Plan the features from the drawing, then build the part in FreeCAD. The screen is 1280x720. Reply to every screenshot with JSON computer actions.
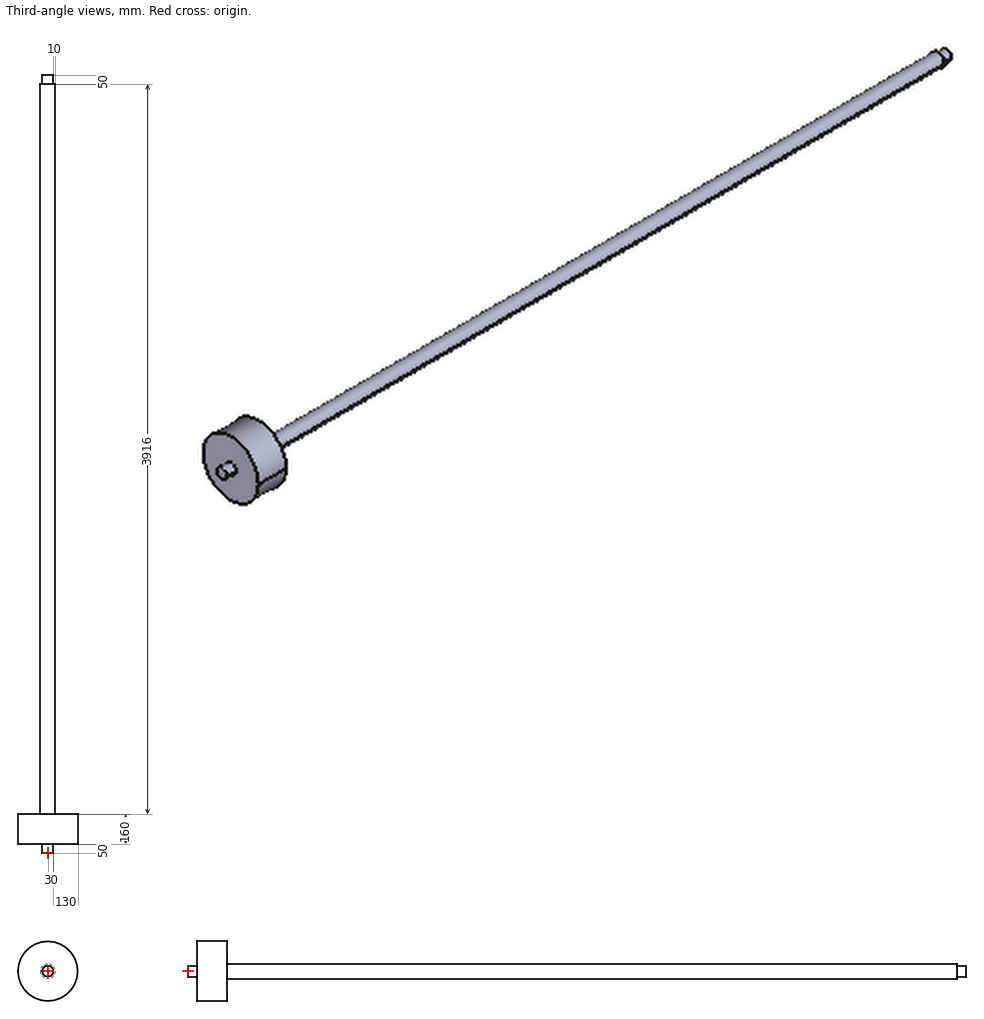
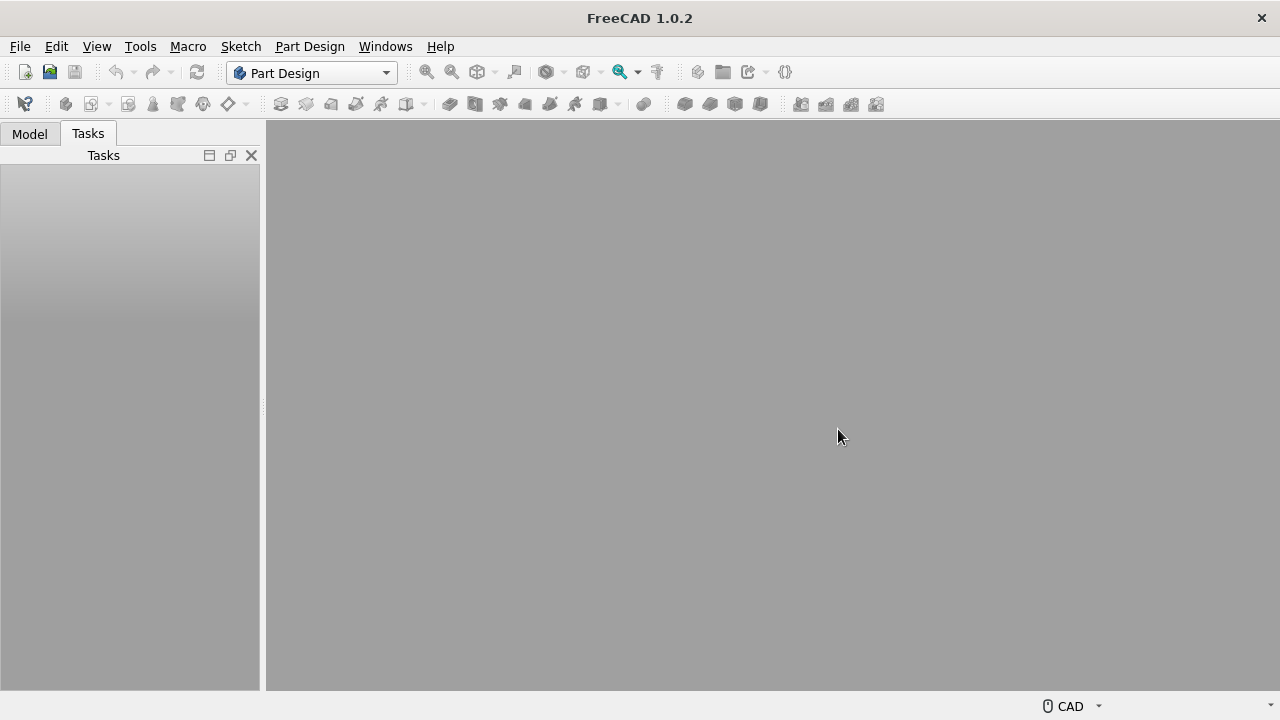
{"action": "left_click", "coordinate": [25, 72]}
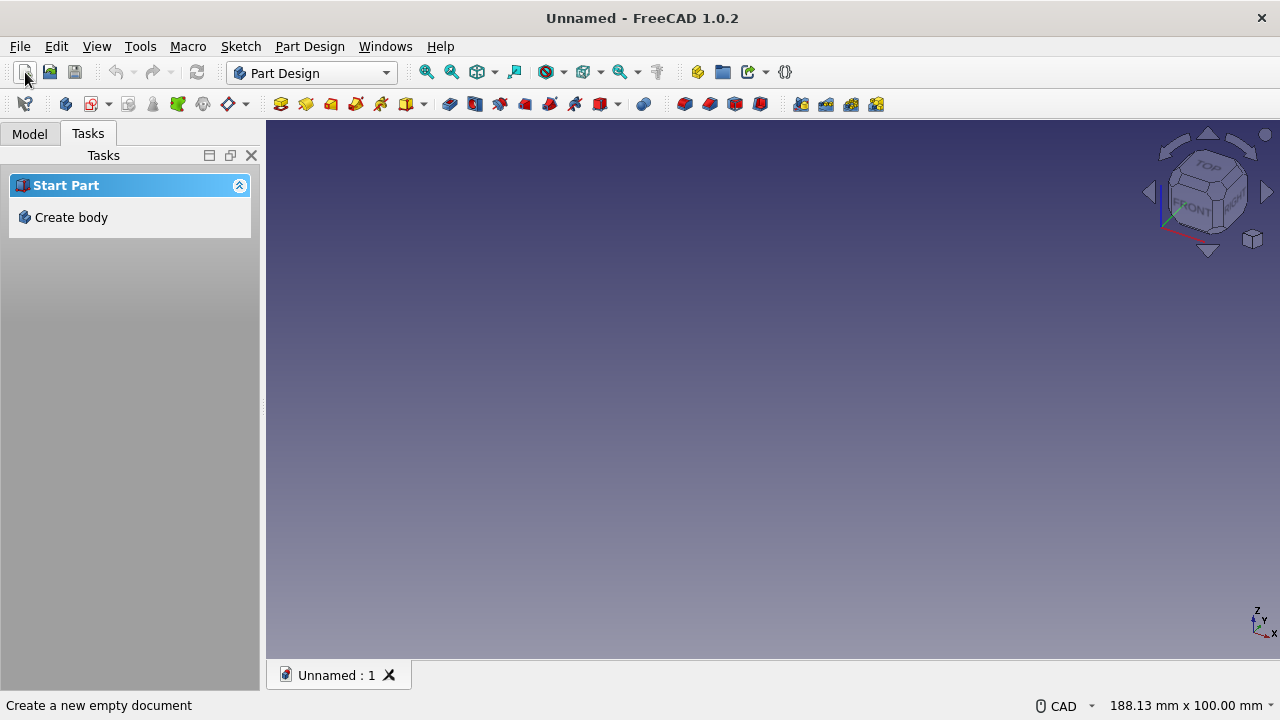
{"action": "left_click", "coordinate": [90, 104]}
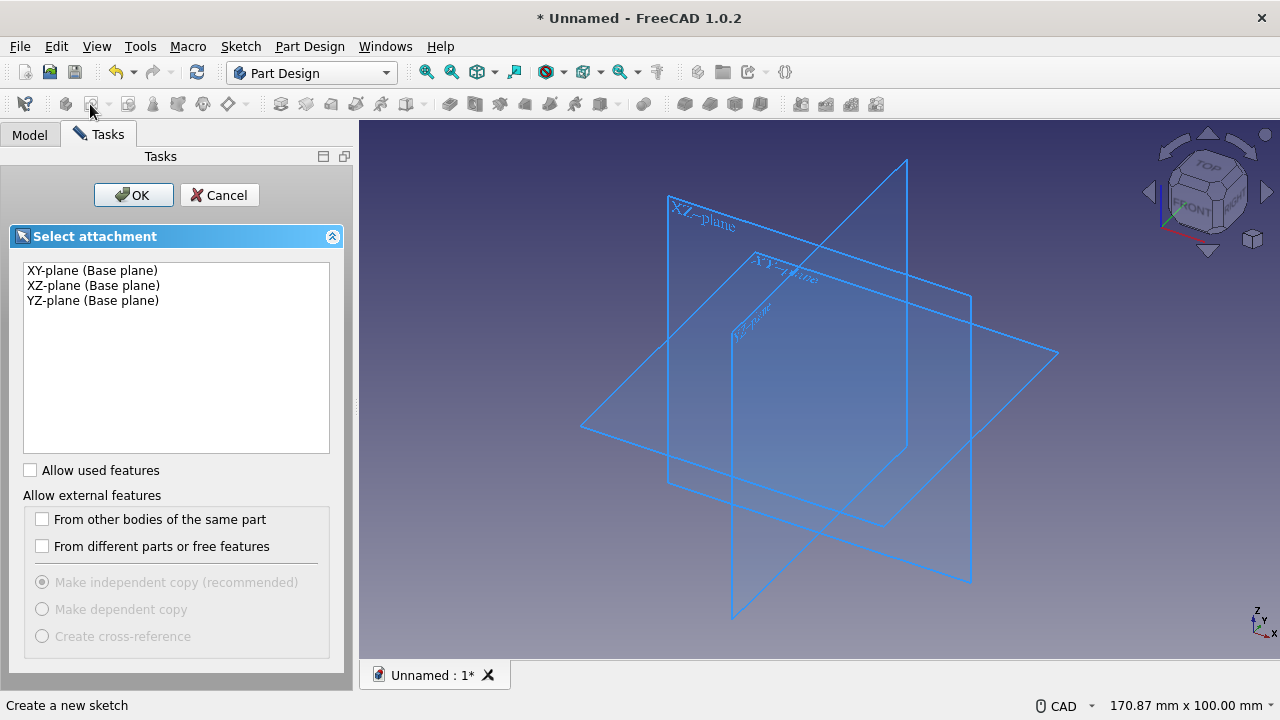
{"action": "left_click", "coordinate": [84, 270]}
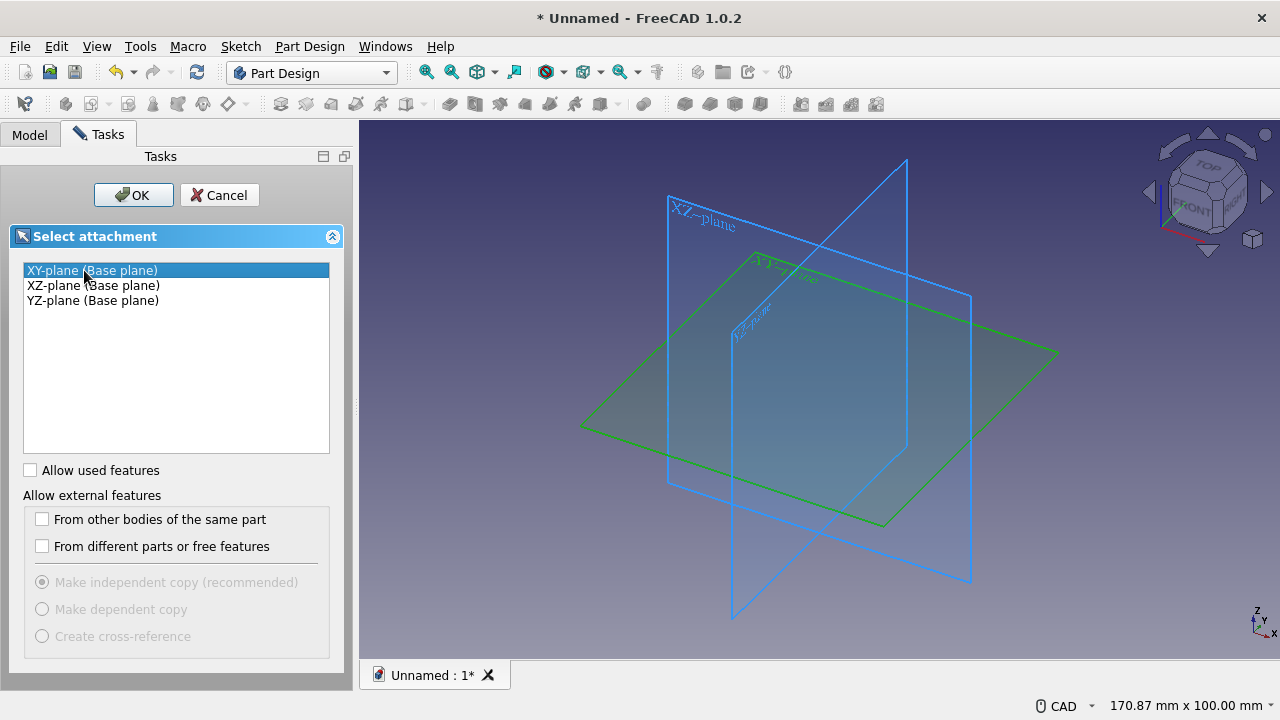
{"action": "left_click", "coordinate": [134, 195]}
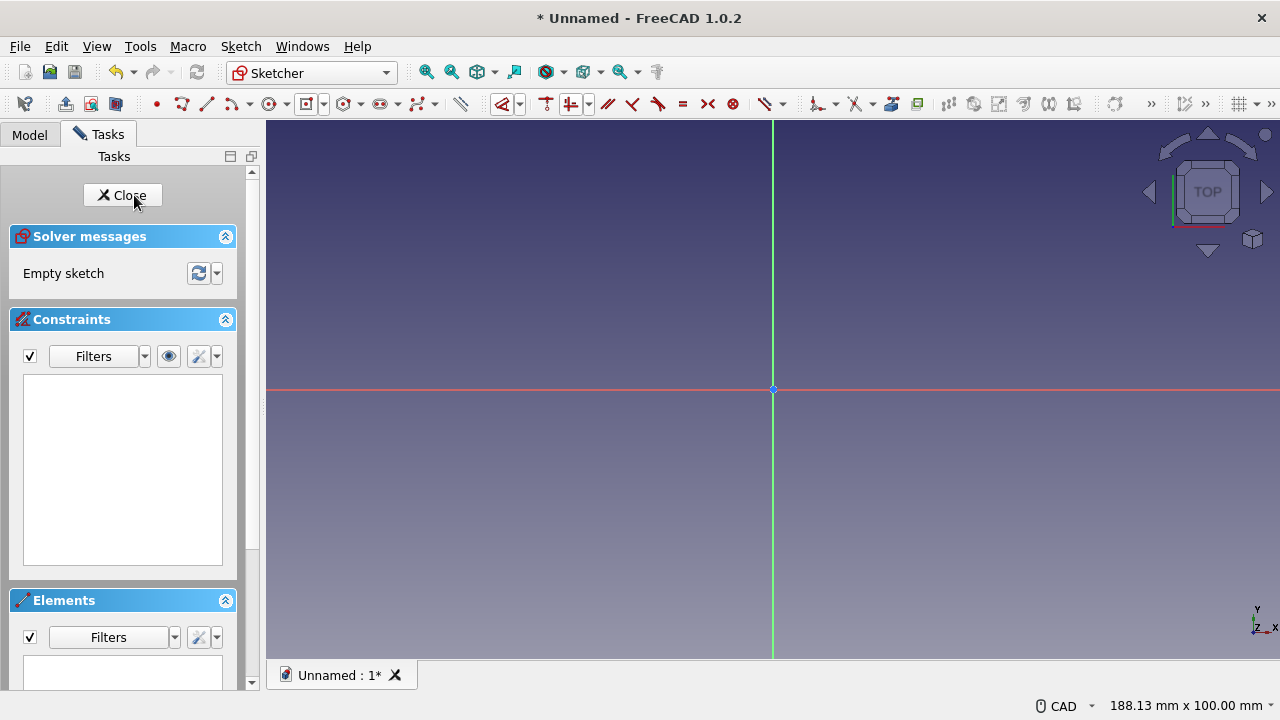
{"action": "scroll", "coordinate": [704, 390], "scroll_direction": "down", "scroll_amount": 15}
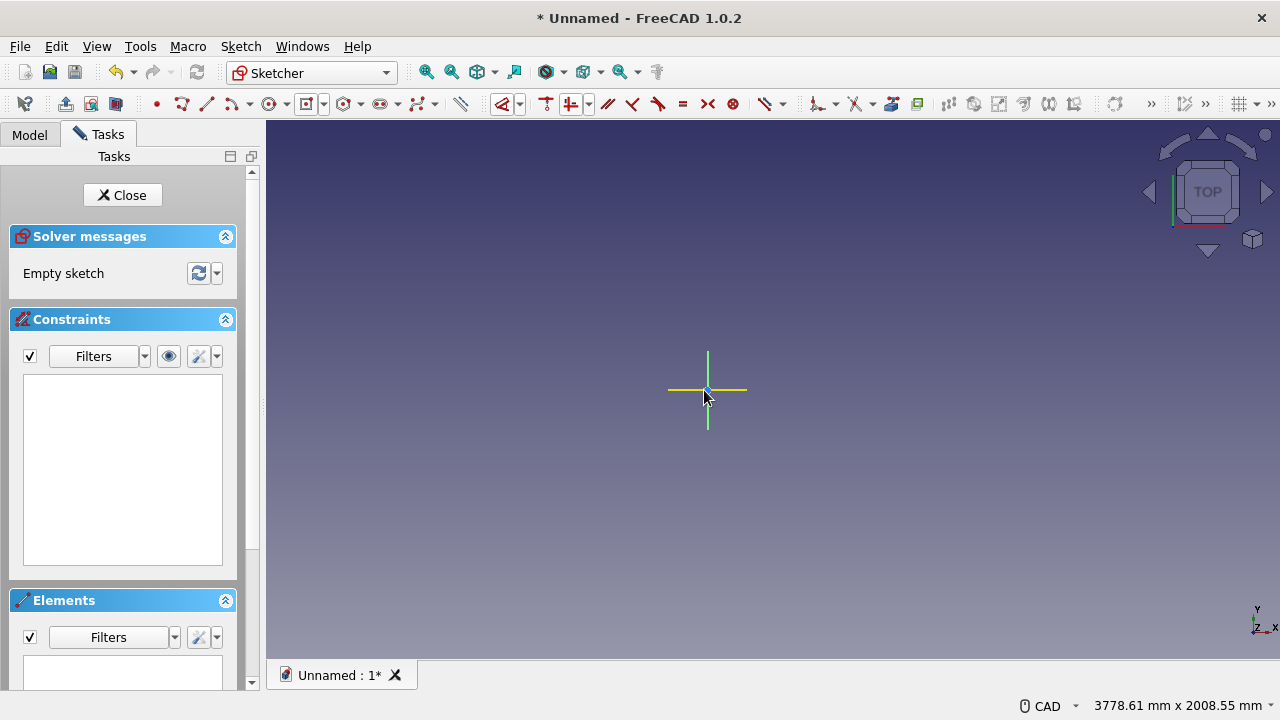
{"action": "scroll", "coordinate": [694, 631], "scroll_direction": "down", "scroll_amount": 6}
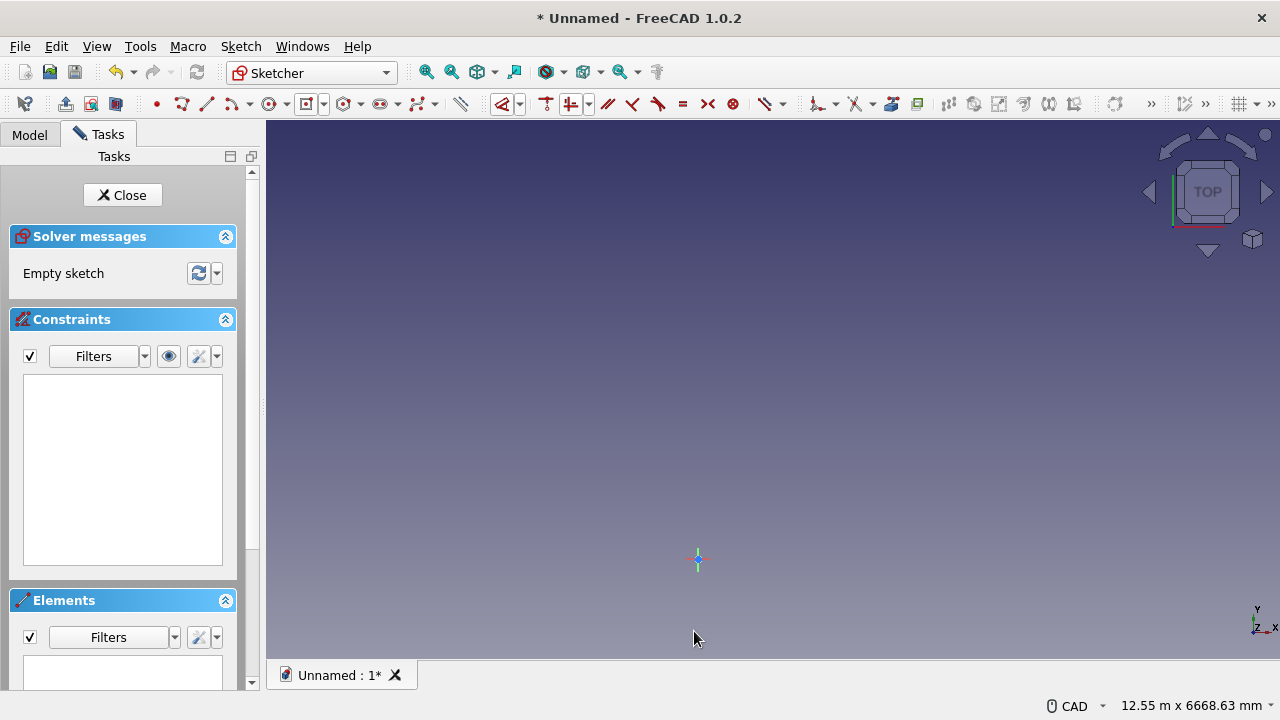
{"action": "left_click", "coordinate": [182, 104]}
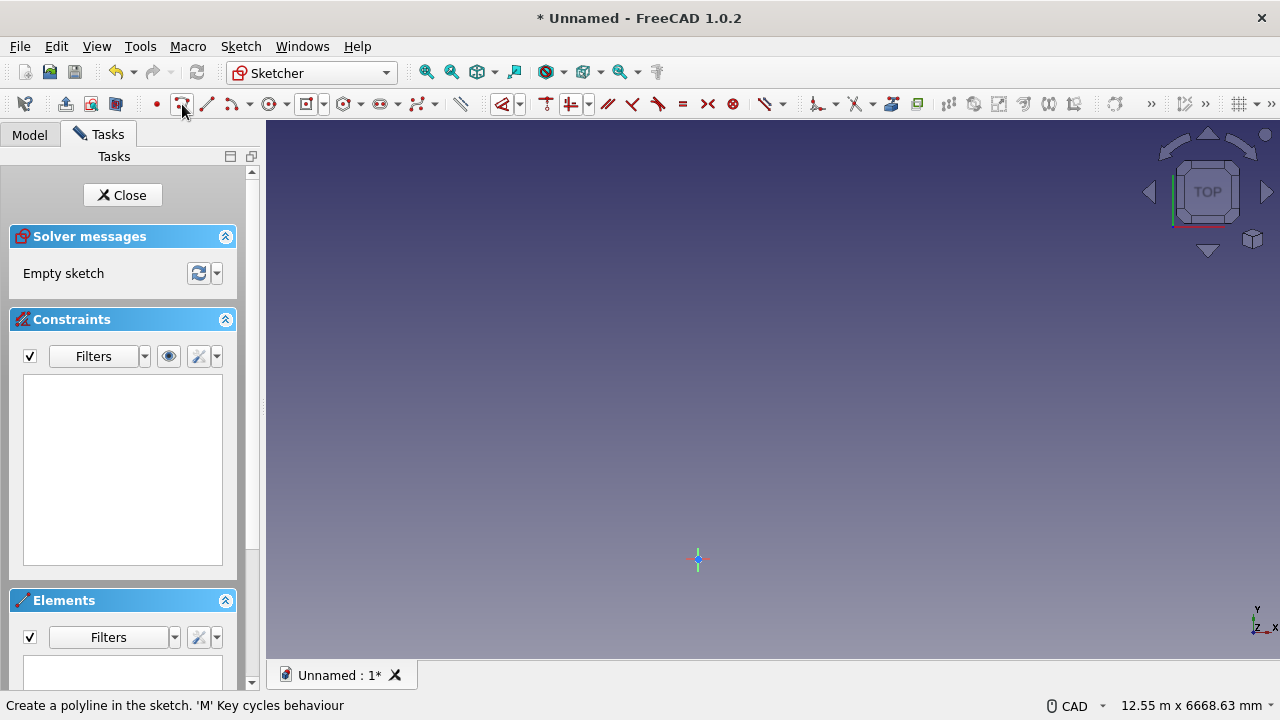
{"action": "left_click", "coordinate": [698, 559]}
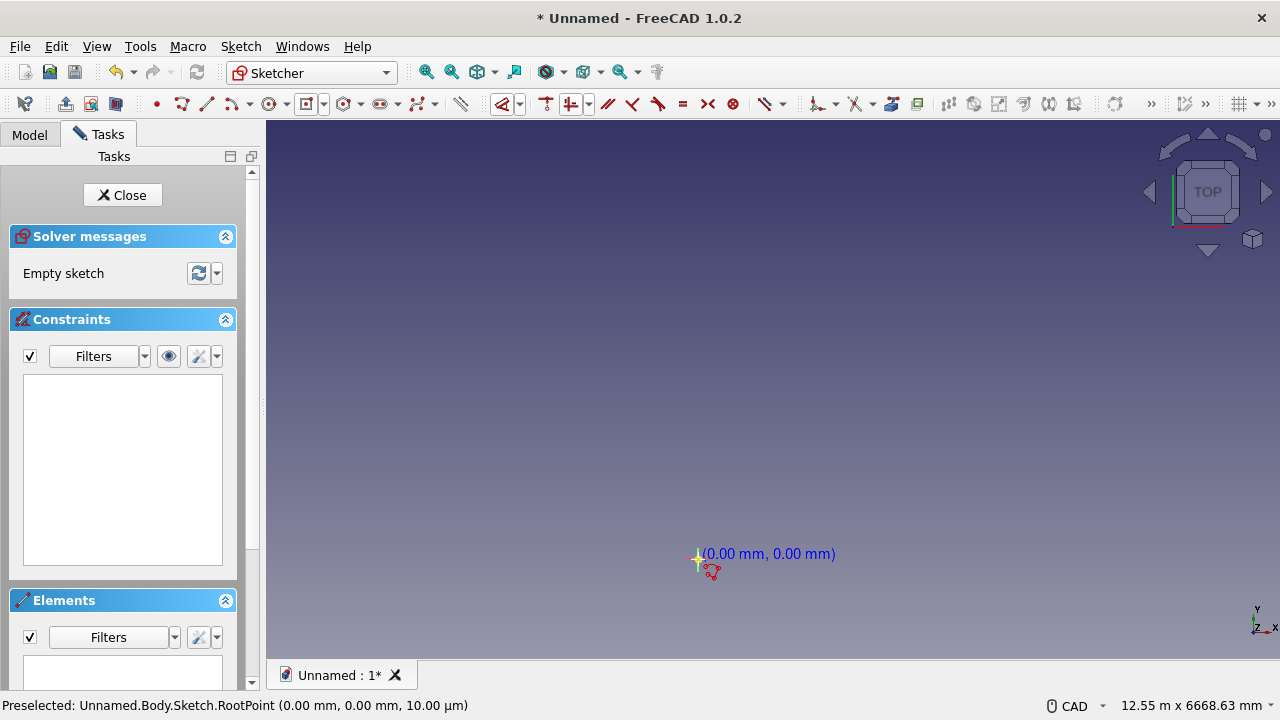
{"action": "scroll", "coordinate": [701, 559], "scroll_direction": "up", "scroll_amount": 10}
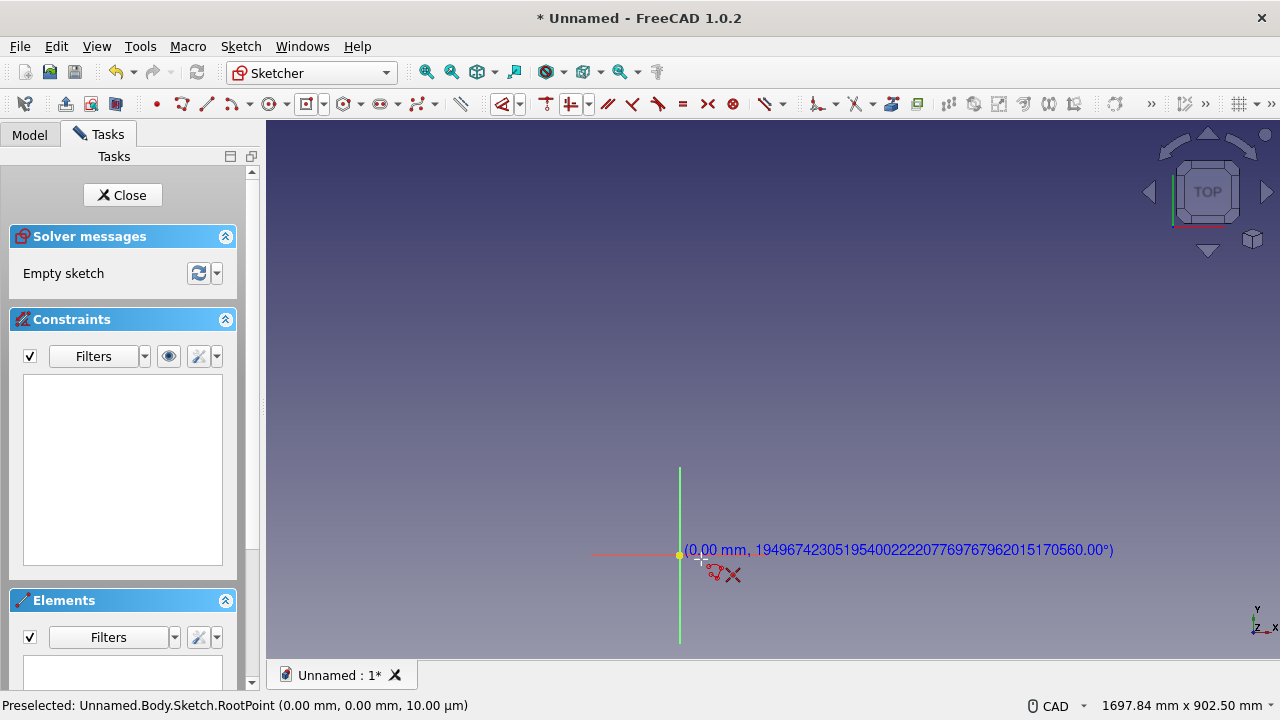
{"action": "left_click", "coordinate": [697, 546]}
{"action": "left_click", "coordinate": [697, 525]}
{"action": "left_click", "coordinate": [775, 525]}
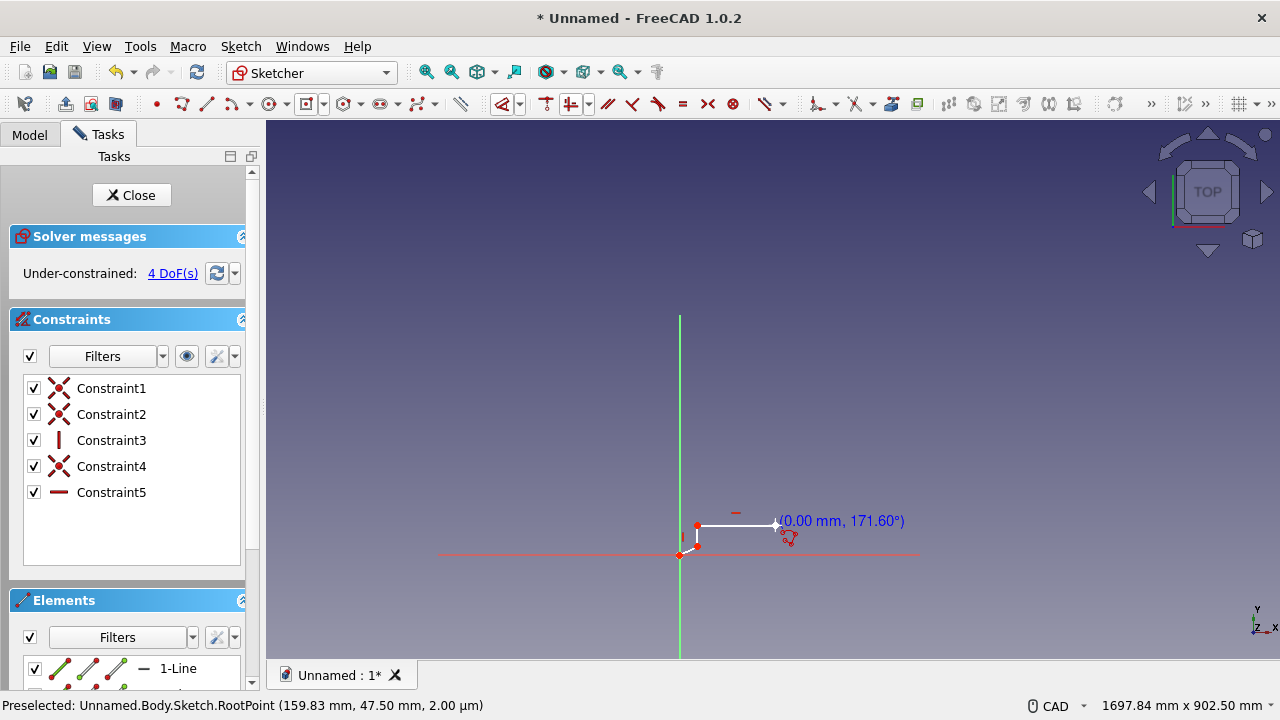
{"action": "scroll", "coordinate": [701, 559], "scroll_direction": "down", "scroll_amount": 10}